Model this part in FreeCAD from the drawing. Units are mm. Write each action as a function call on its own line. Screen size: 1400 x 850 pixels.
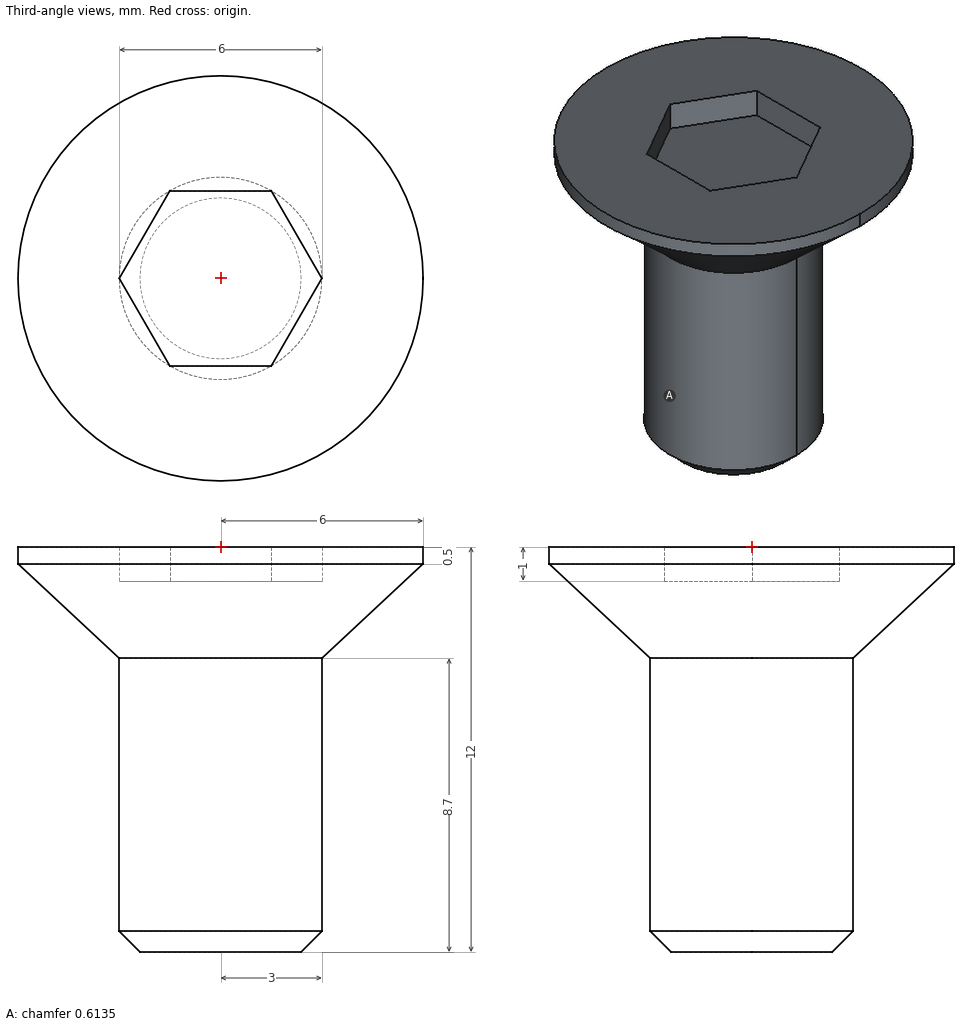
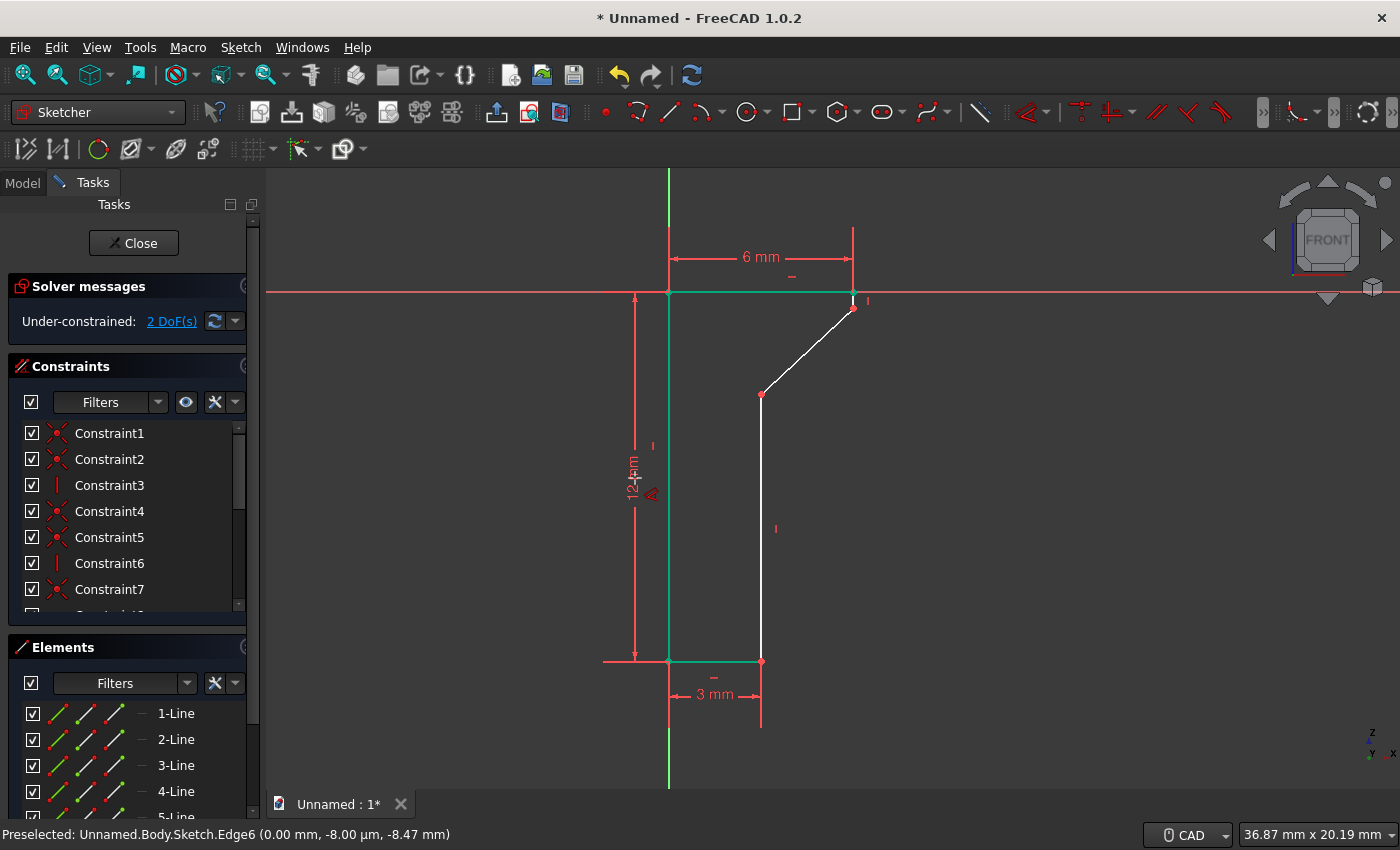
scroll(853, 301, up, 5)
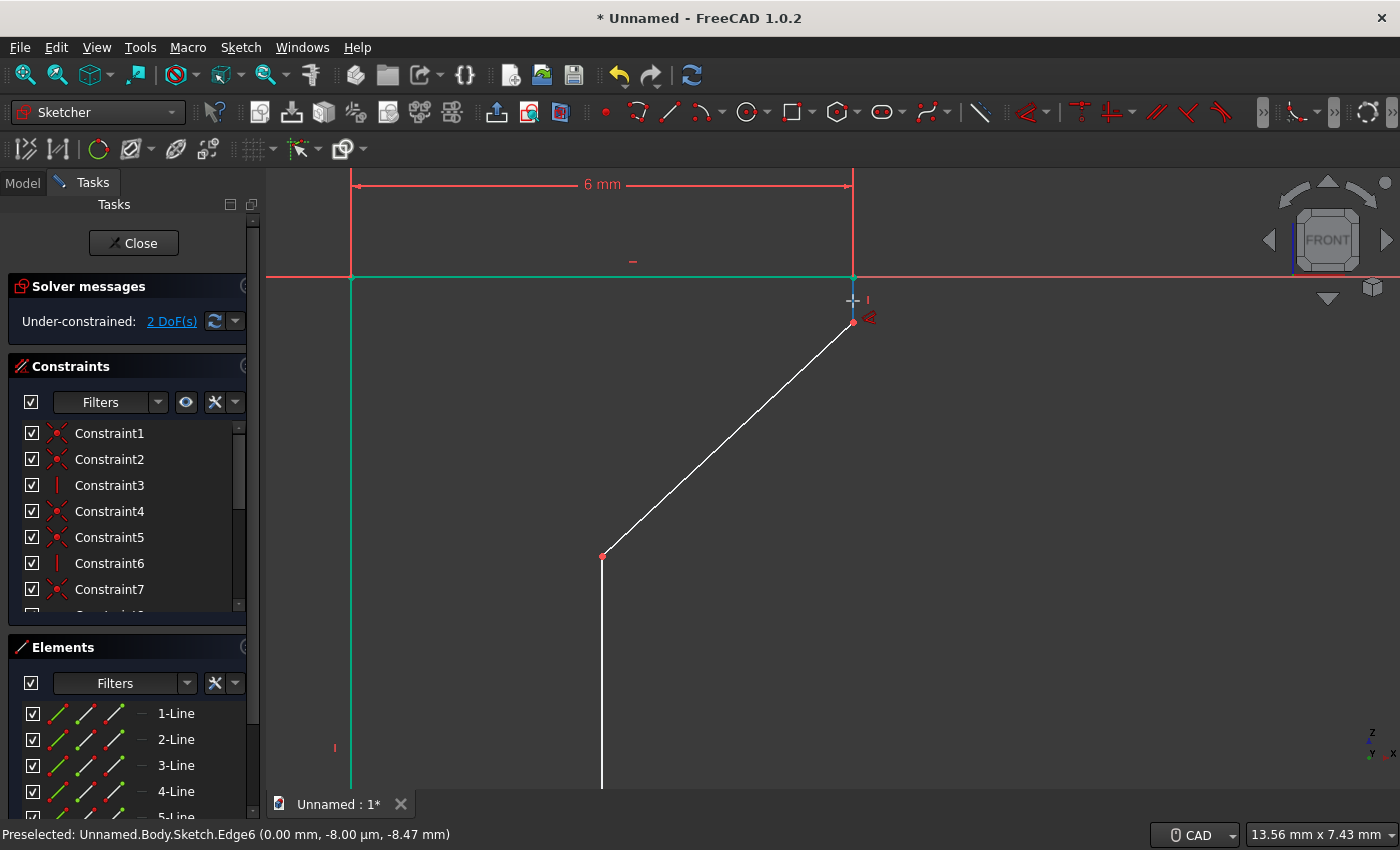
click(853, 300)
click(887, 300)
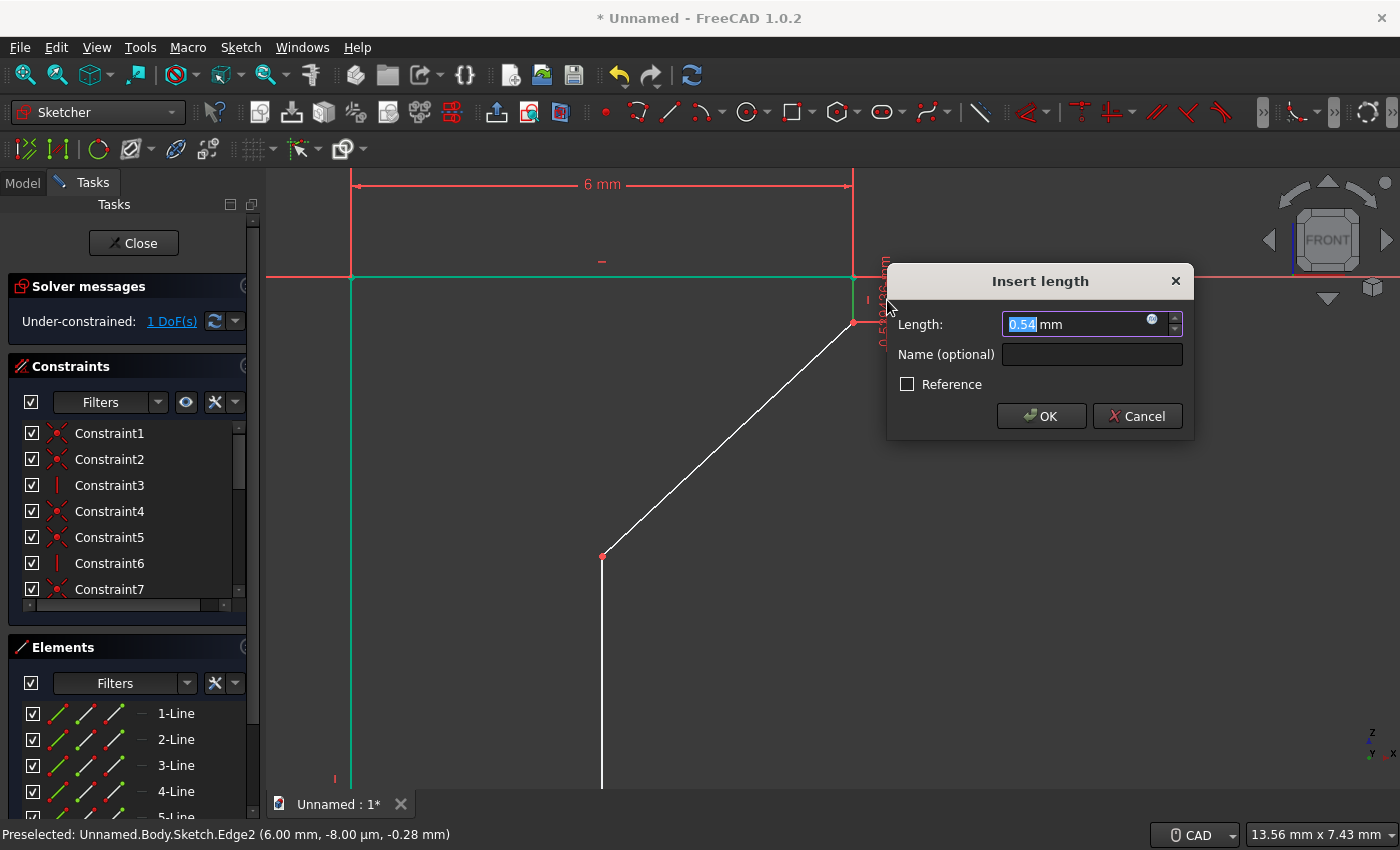
text(0.5)
key(Return)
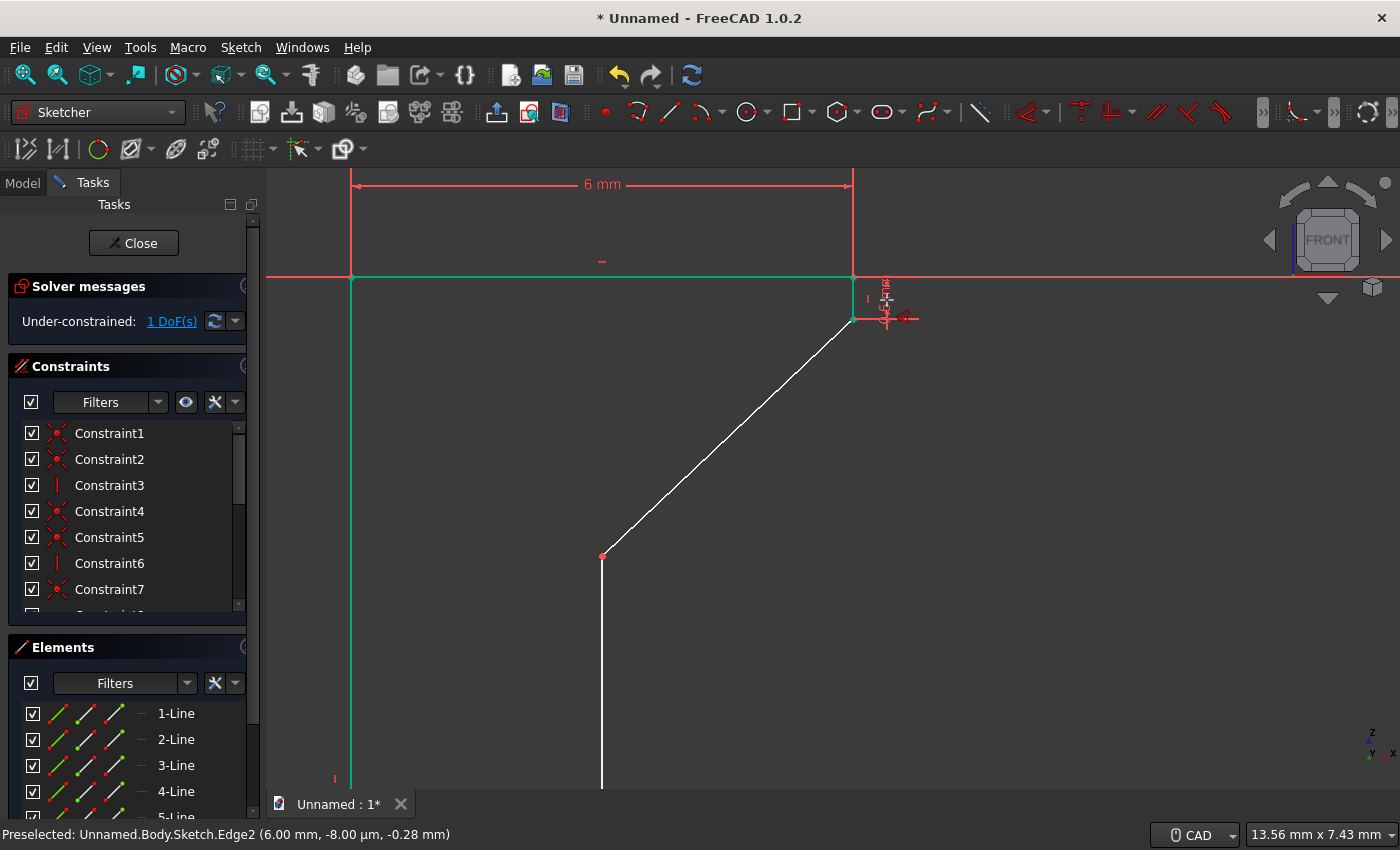
click(602, 701)
click(636, 659)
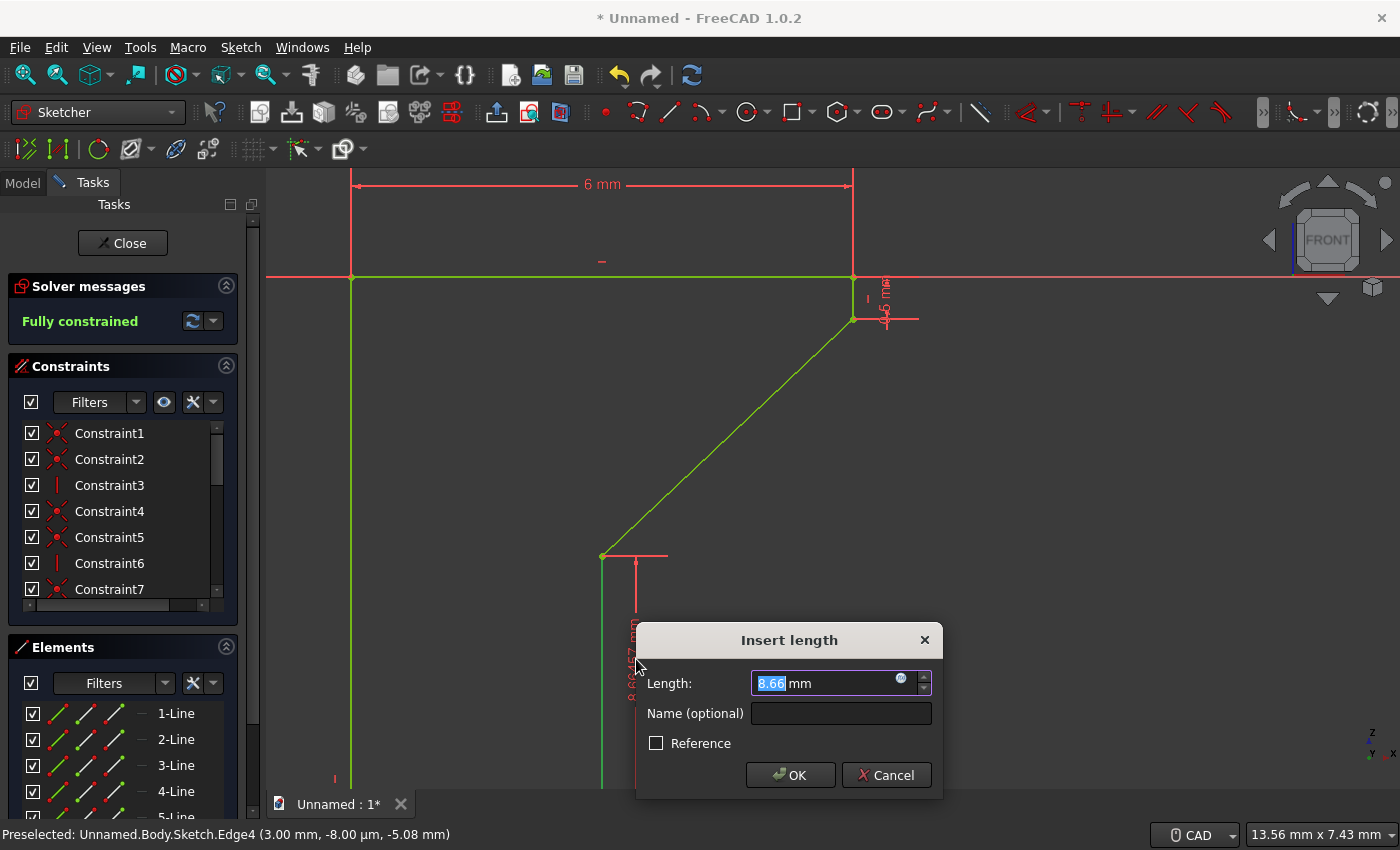
text(8.7)
key(Return)
key(Escape)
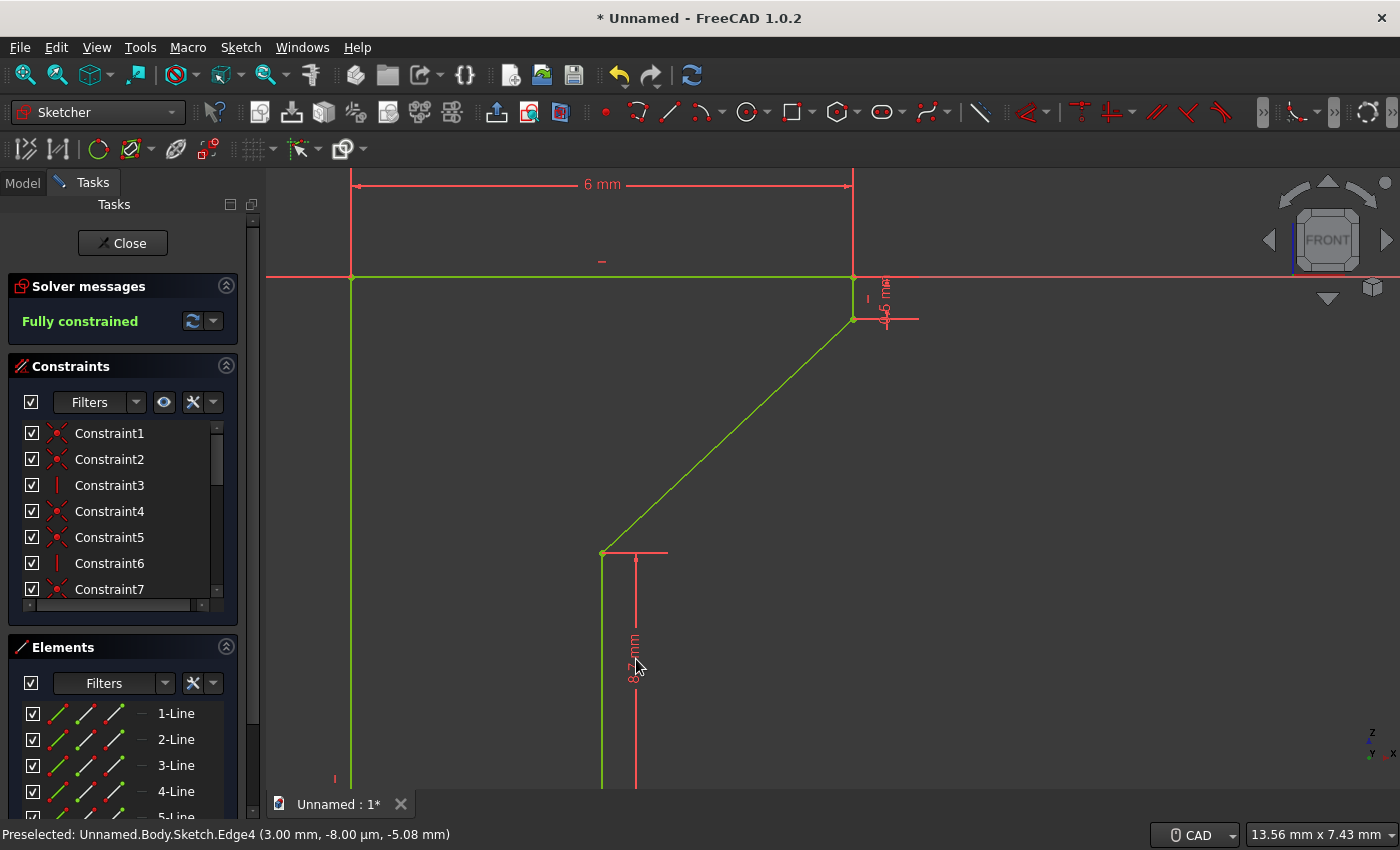
click(123, 243)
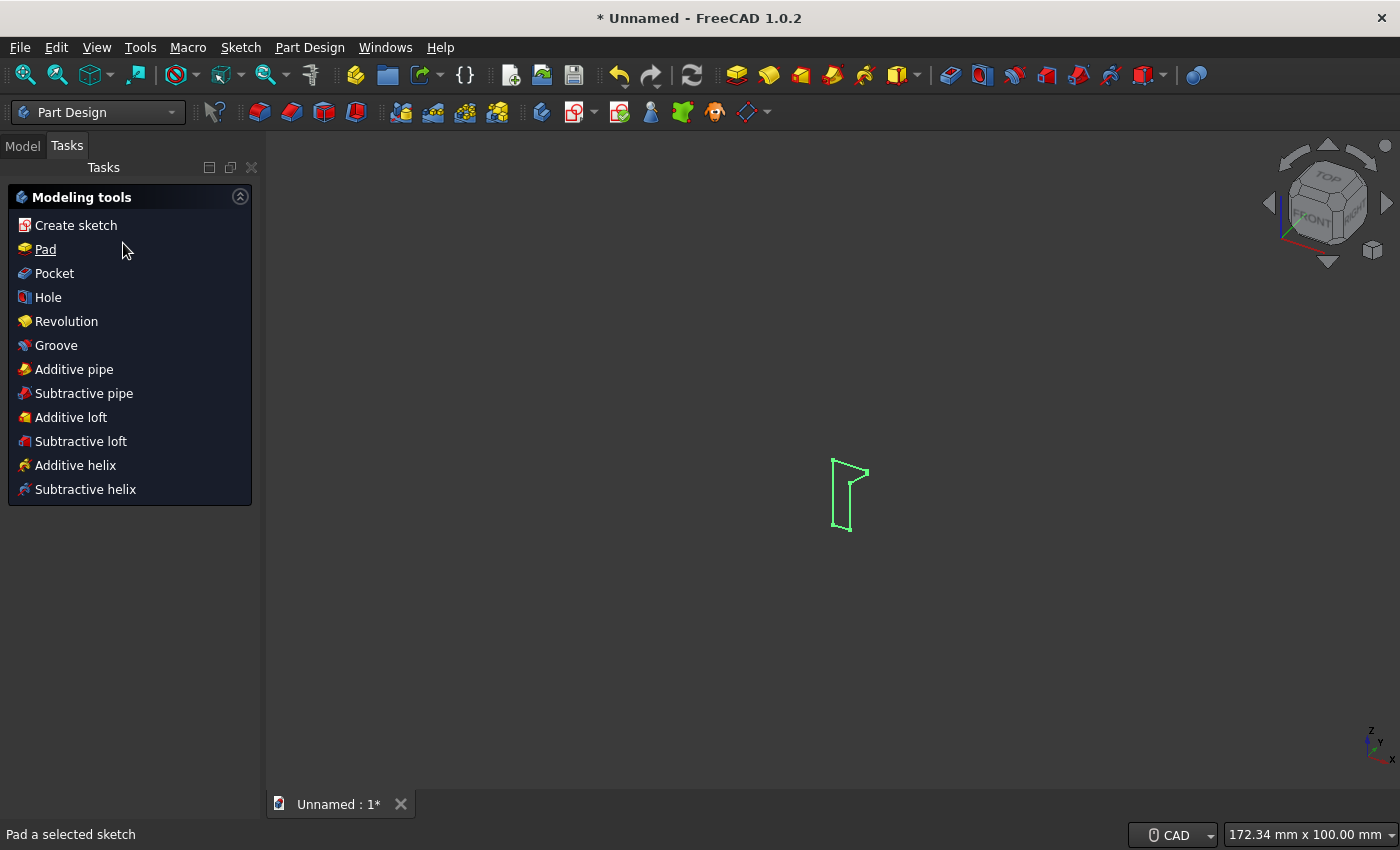
click(770, 76)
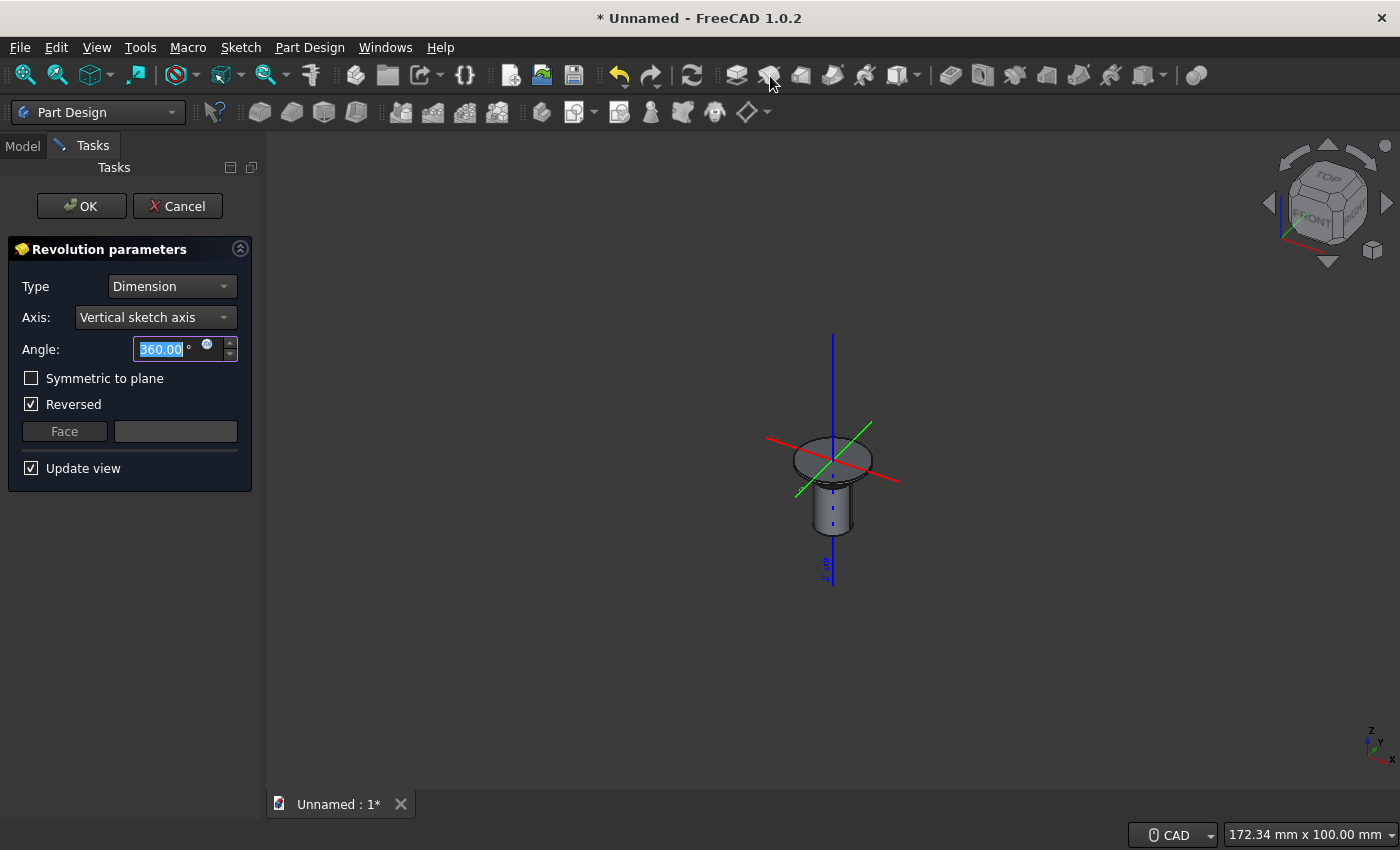
click(82, 206)